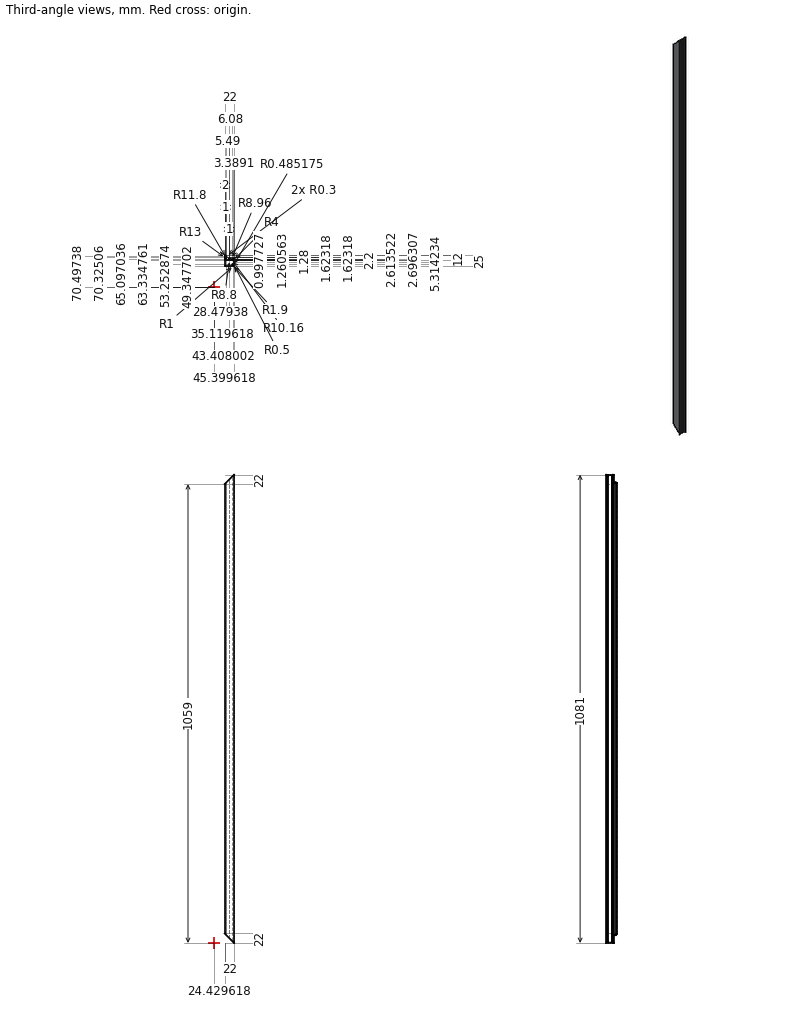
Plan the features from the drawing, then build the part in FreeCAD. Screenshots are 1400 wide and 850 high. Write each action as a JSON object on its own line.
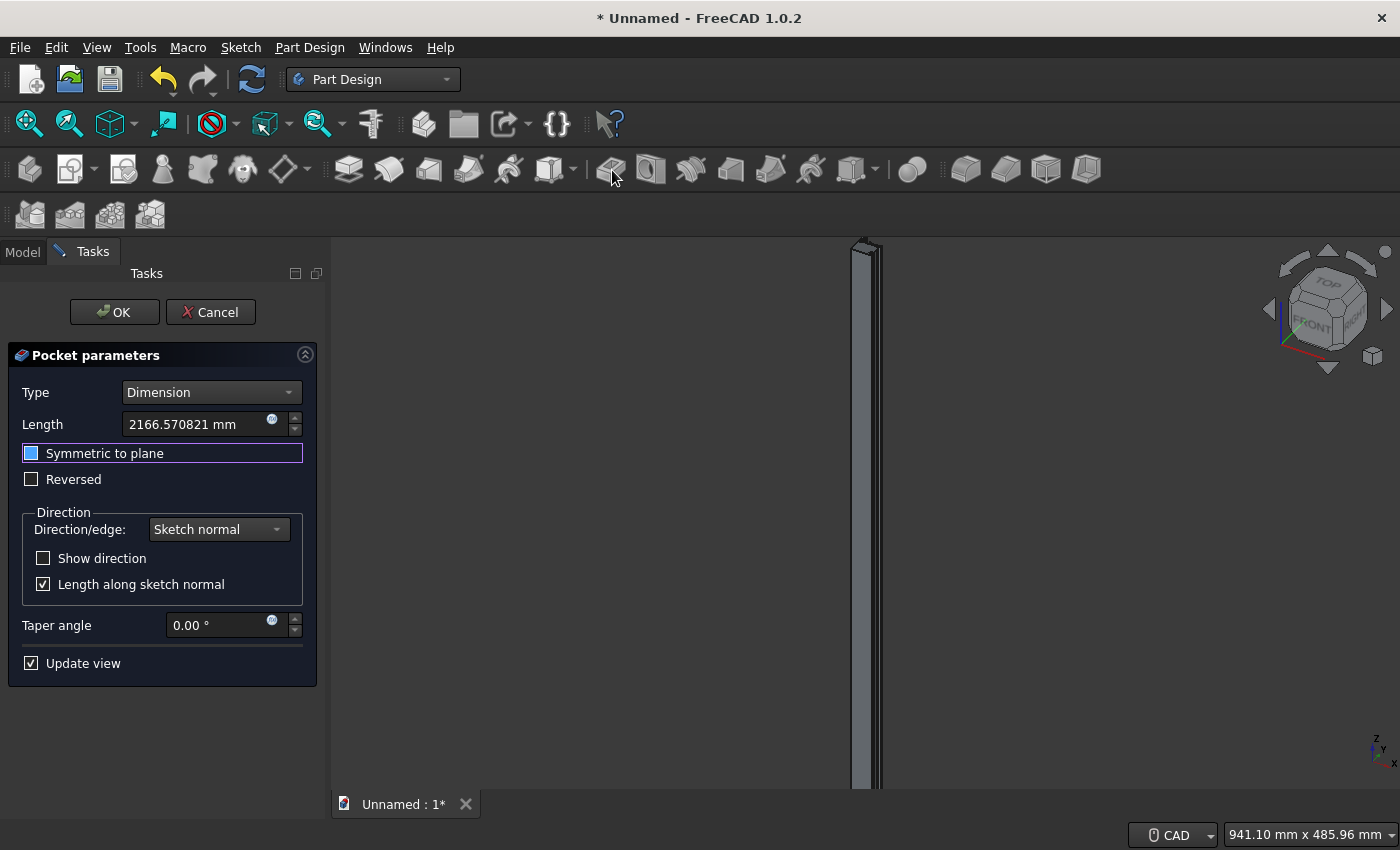
{"action": "left_click", "coordinate": [30, 453]}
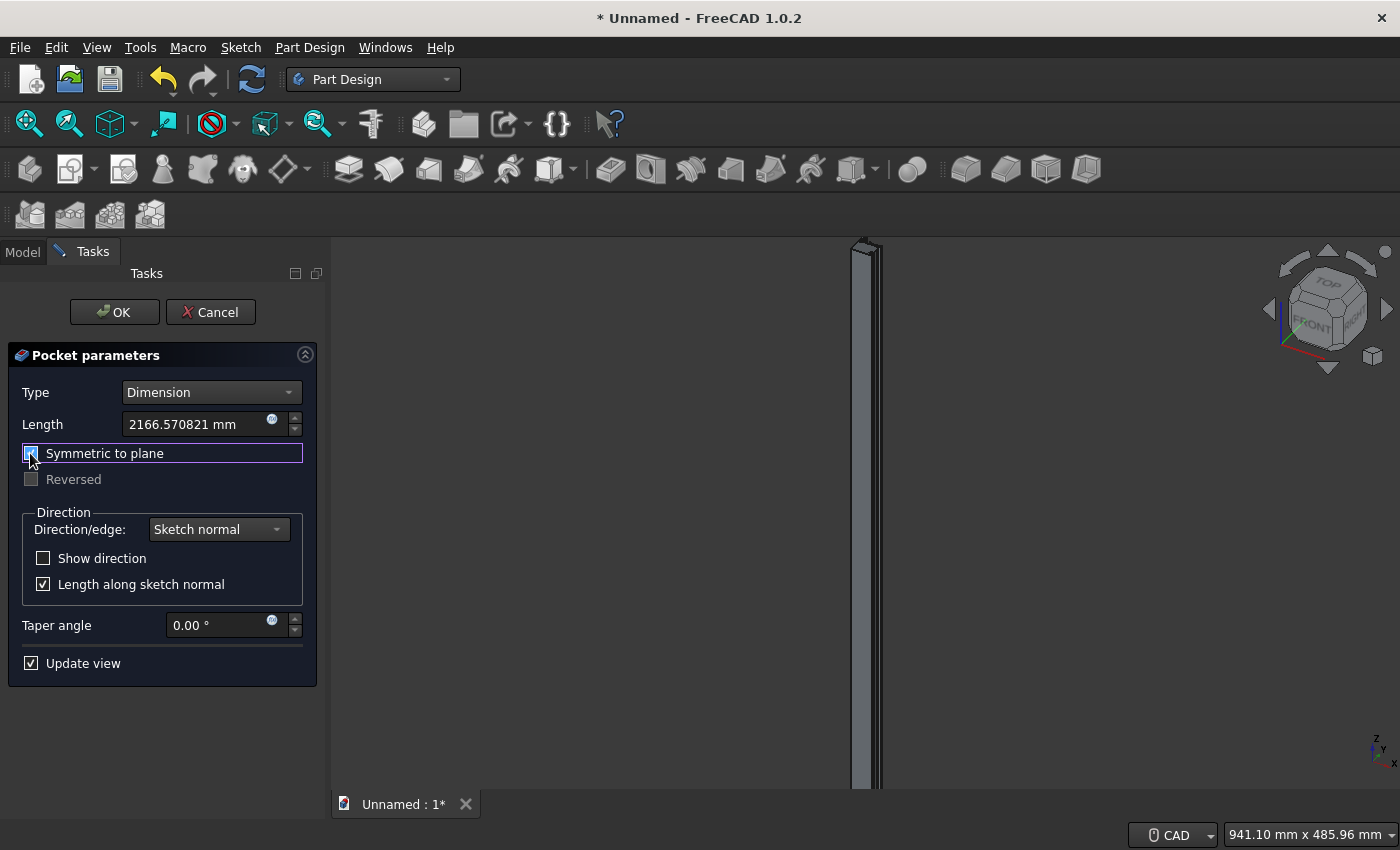
{"action": "left_click", "coordinate": [115, 312]}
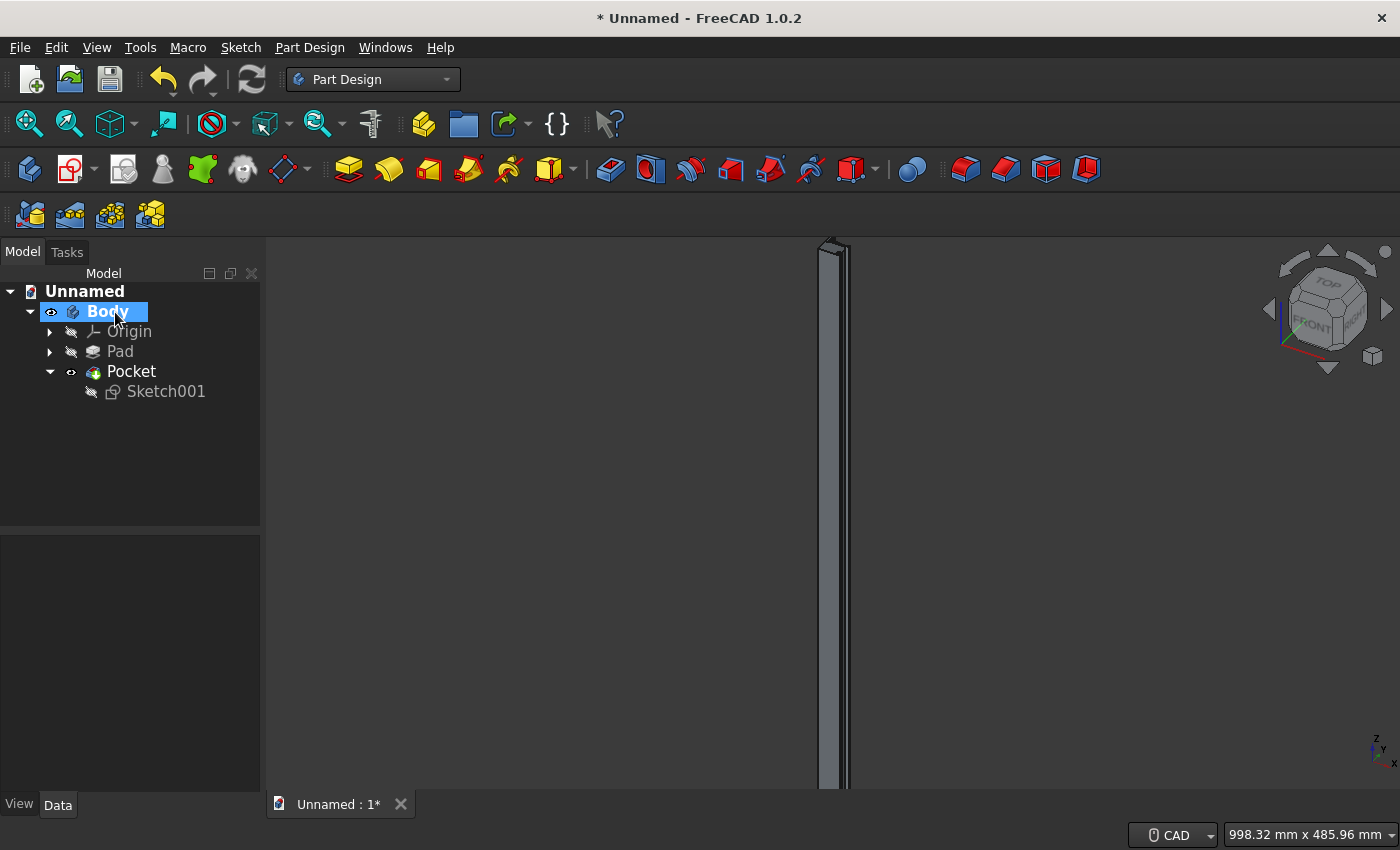
{"action": "left_click", "coordinate": [30, 124]}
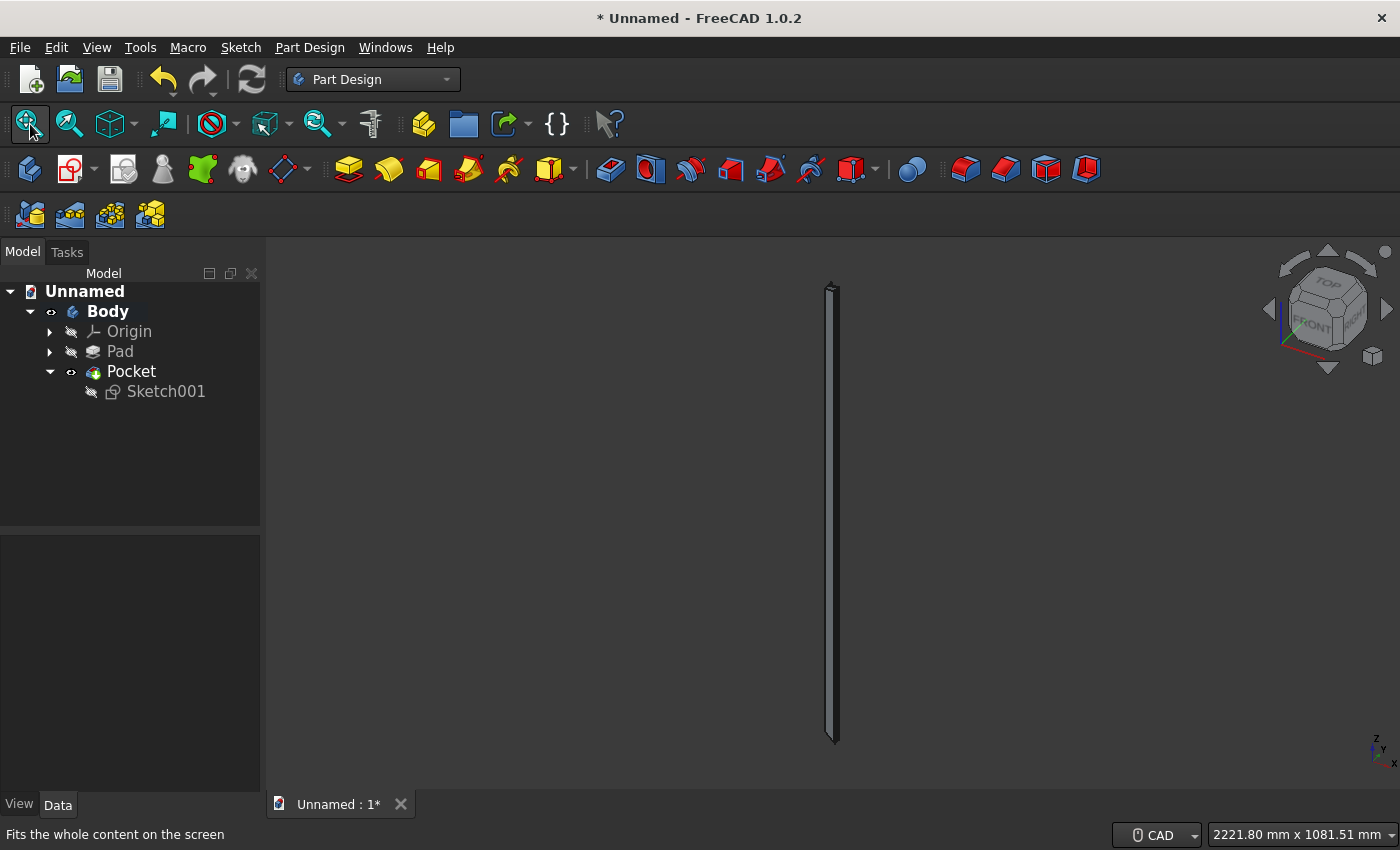
{"action": "scroll", "coordinate": [830, 321], "scroll_direction": "up", "scroll_amount": 4}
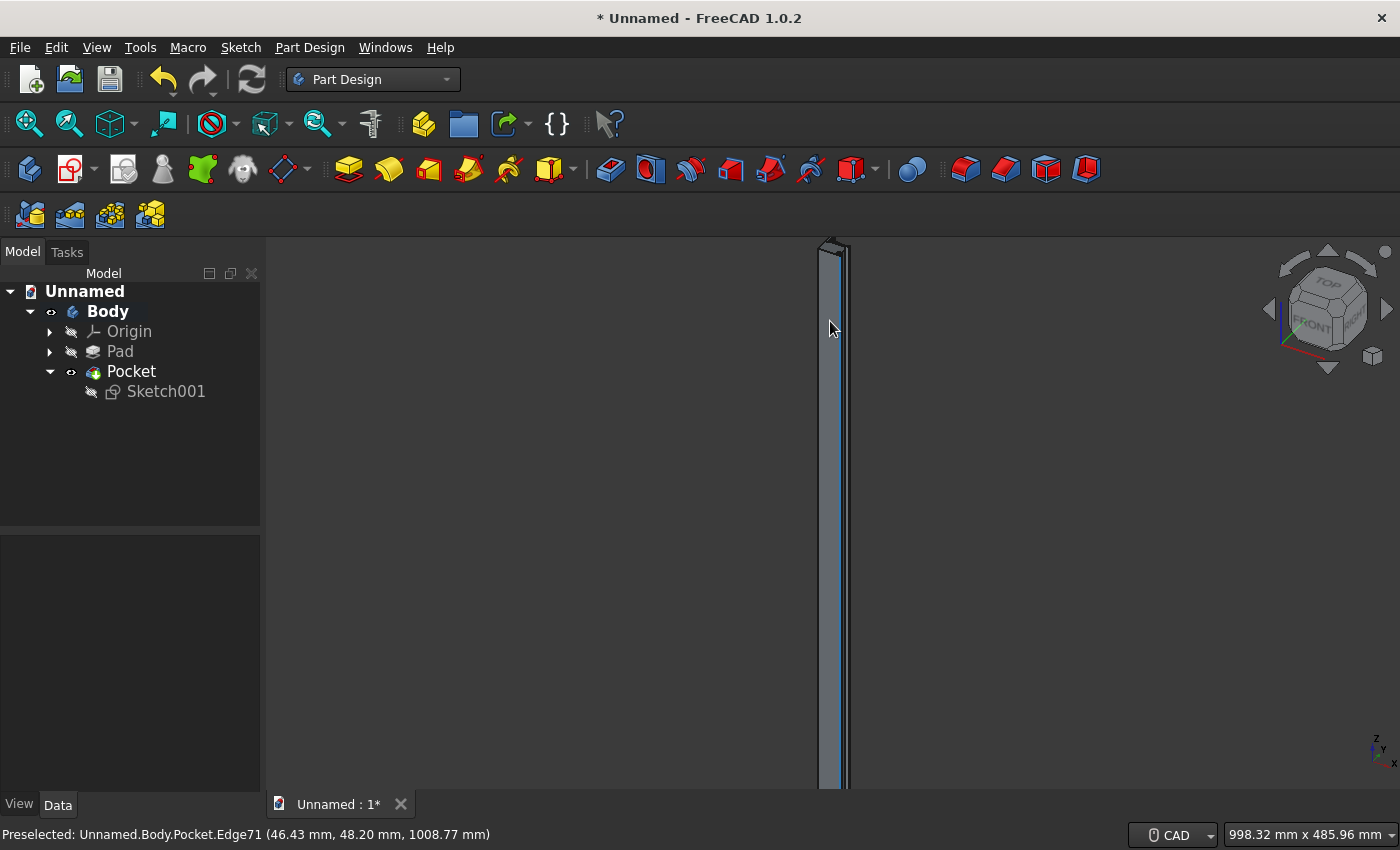
{"action": "left_click", "coordinate": [829, 323]}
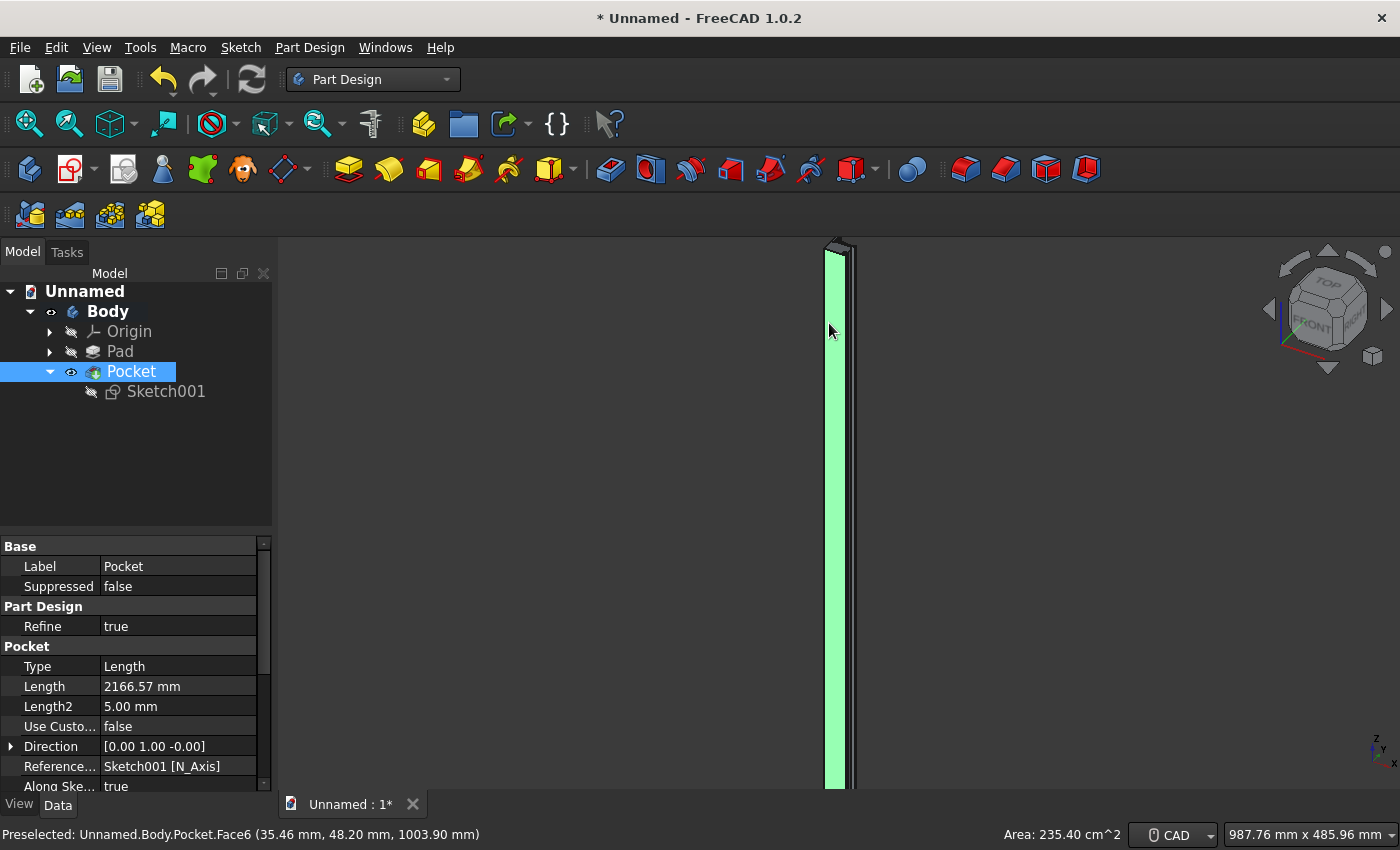
{"action": "left_click", "coordinate": [70, 170]}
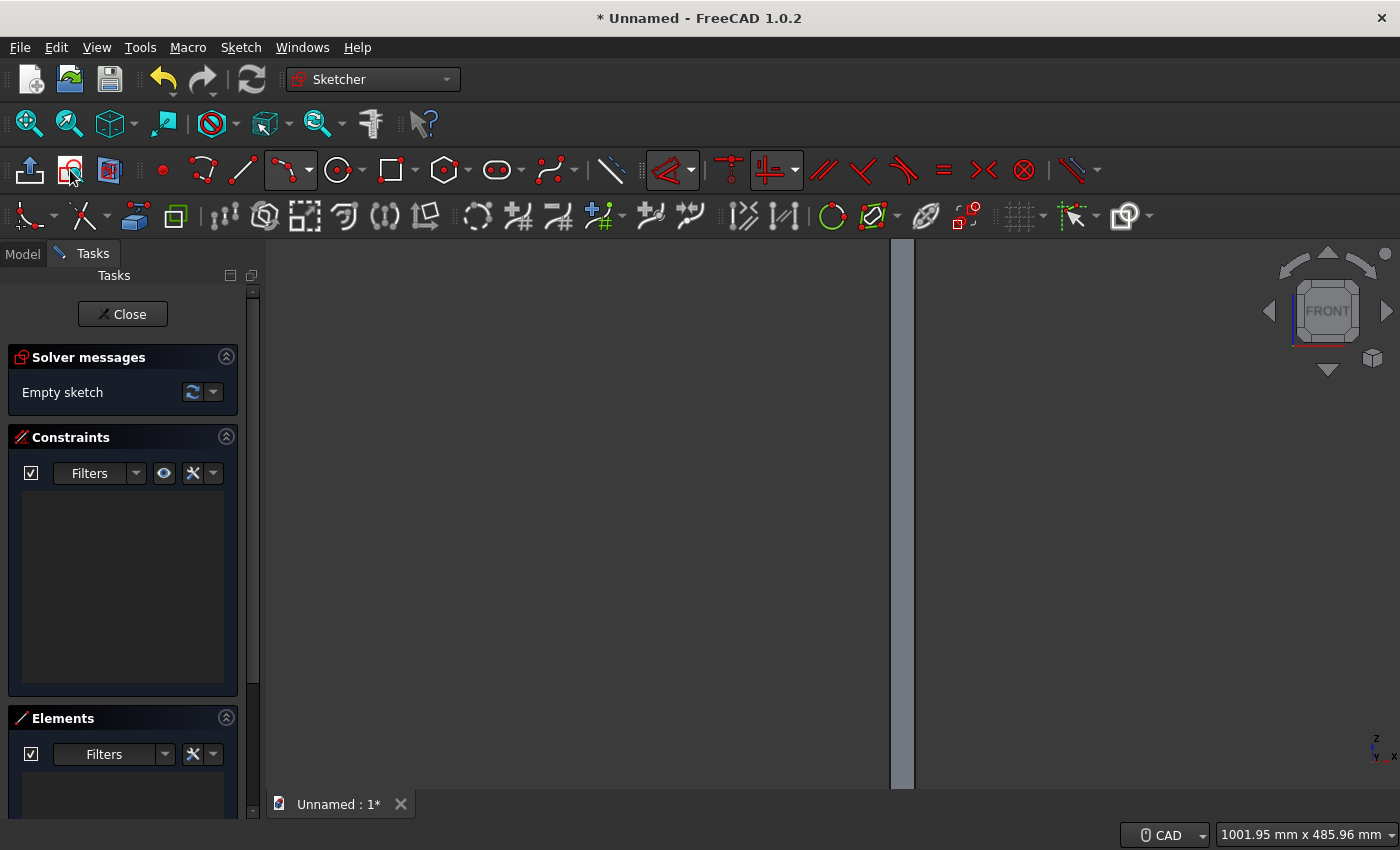
{"action": "scroll", "coordinate": [764, 514], "scroll_direction": "down", "scroll_amount": 5}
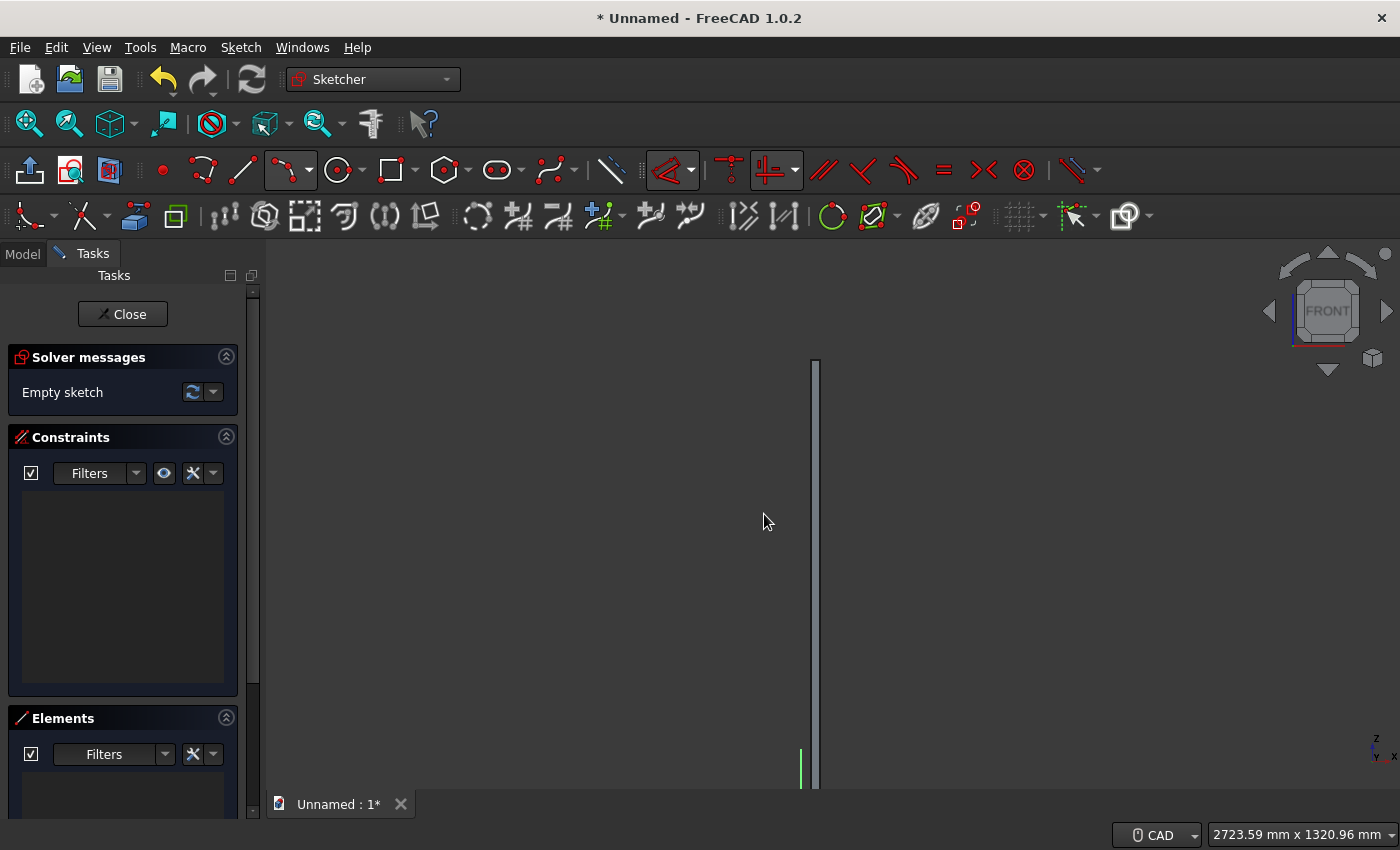
{"action": "scroll", "coordinate": [818, 357], "scroll_direction": "up", "scroll_amount": 15}